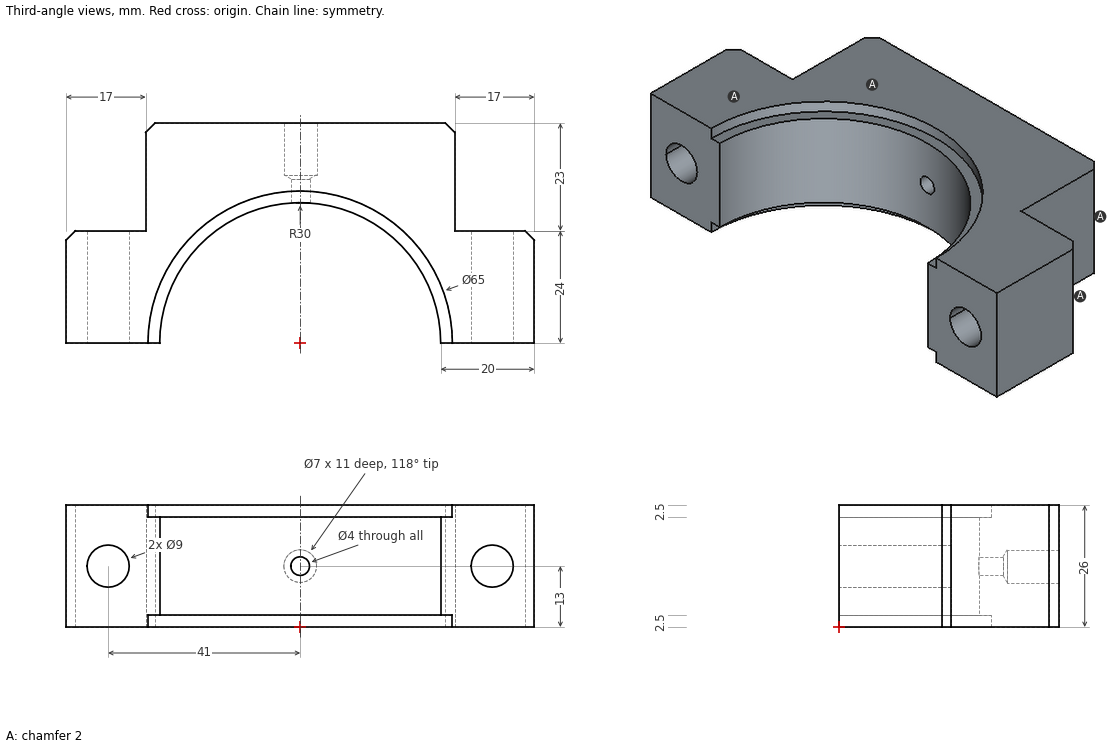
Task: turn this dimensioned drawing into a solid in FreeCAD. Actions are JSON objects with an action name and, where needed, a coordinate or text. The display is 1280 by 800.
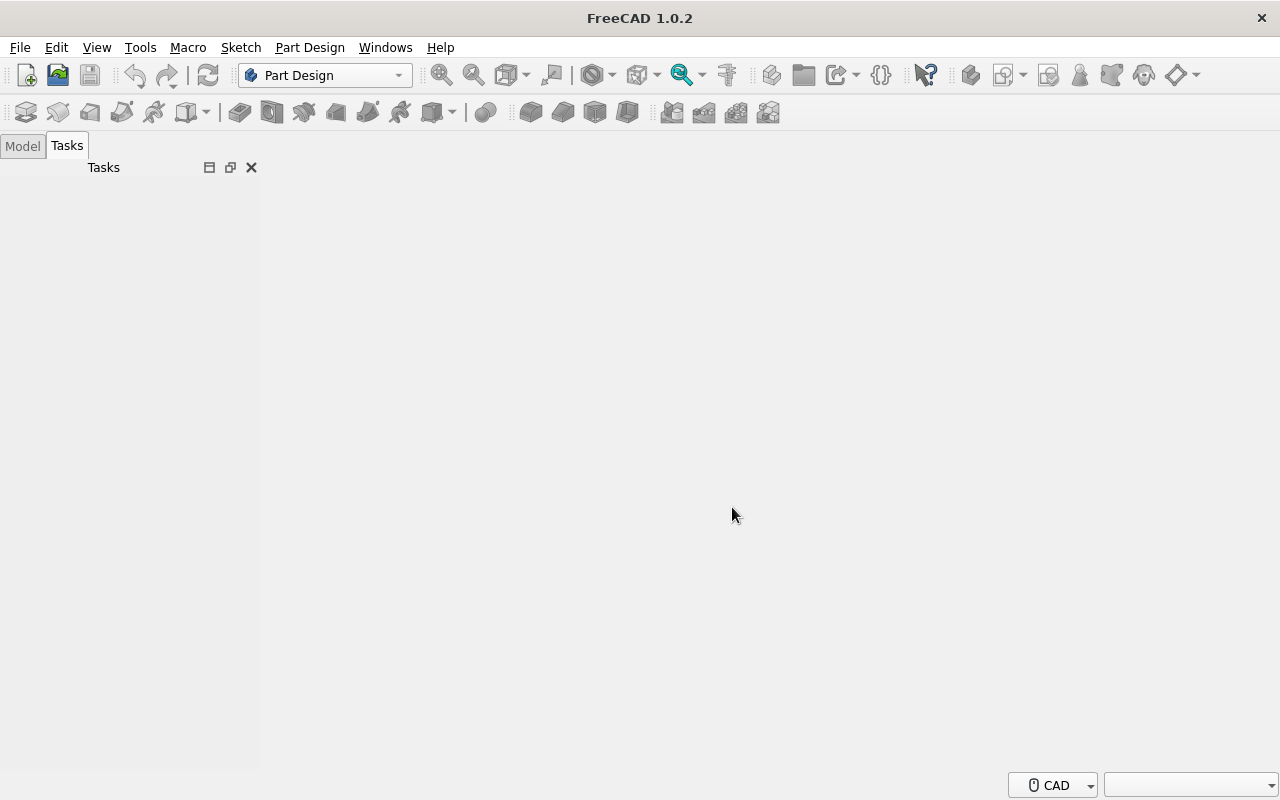
{"action": "key", "text": "ctrl+n"}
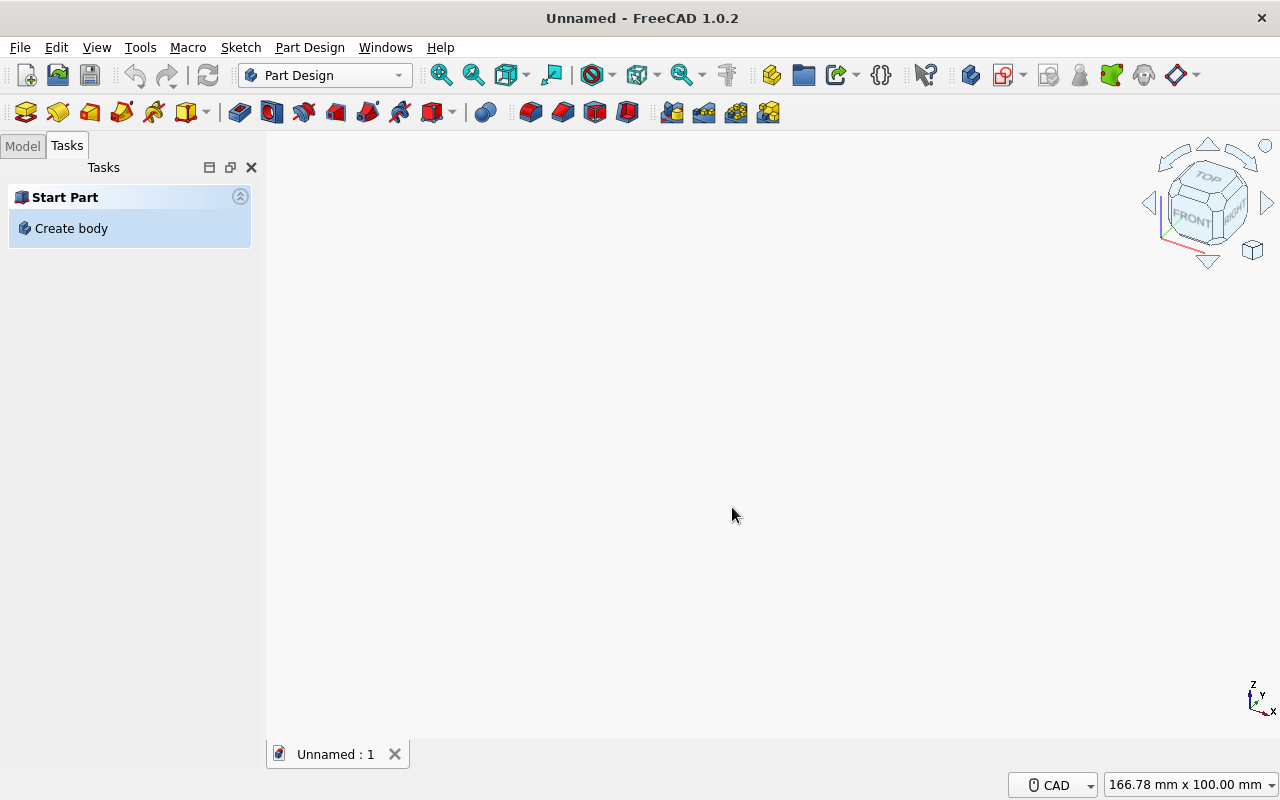
{"action": "left_click", "coordinate": [1004, 76]}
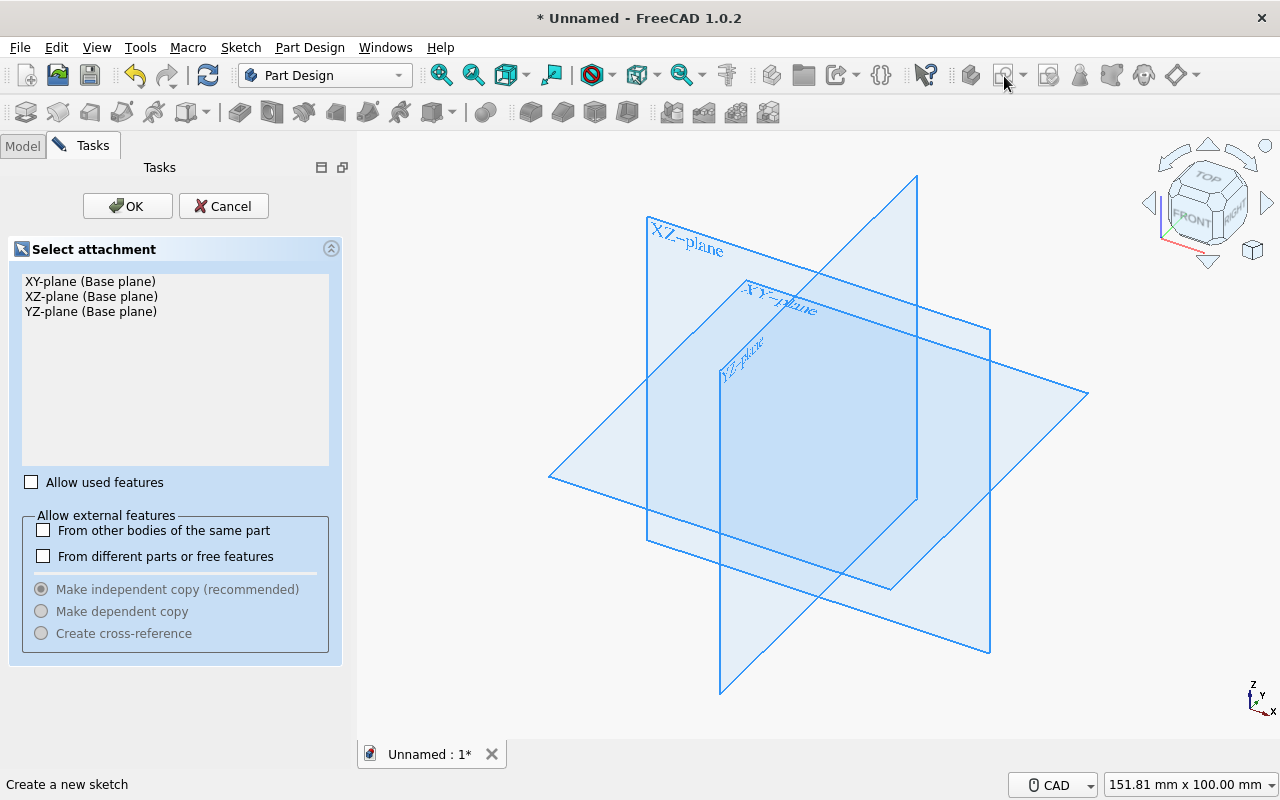
{"action": "left_click", "coordinate": [82, 282]}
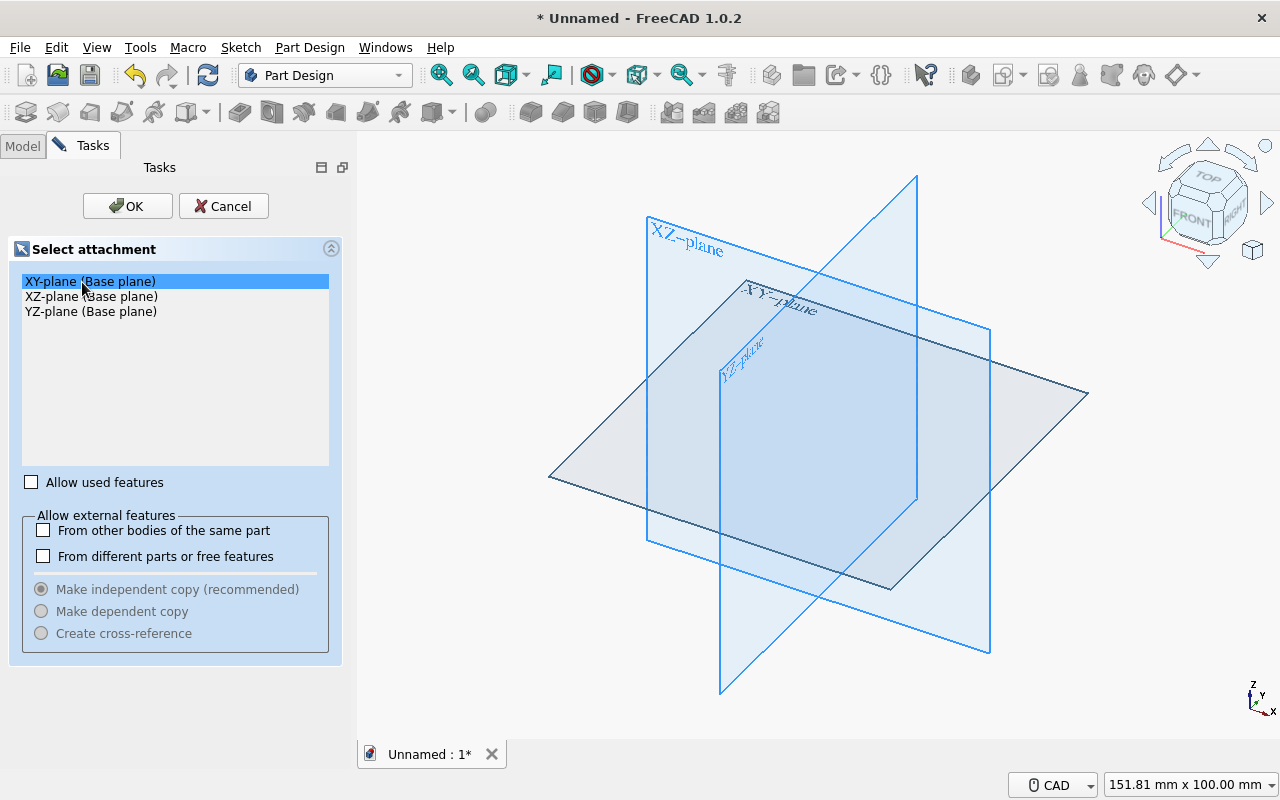
{"action": "left_click", "coordinate": [128, 206]}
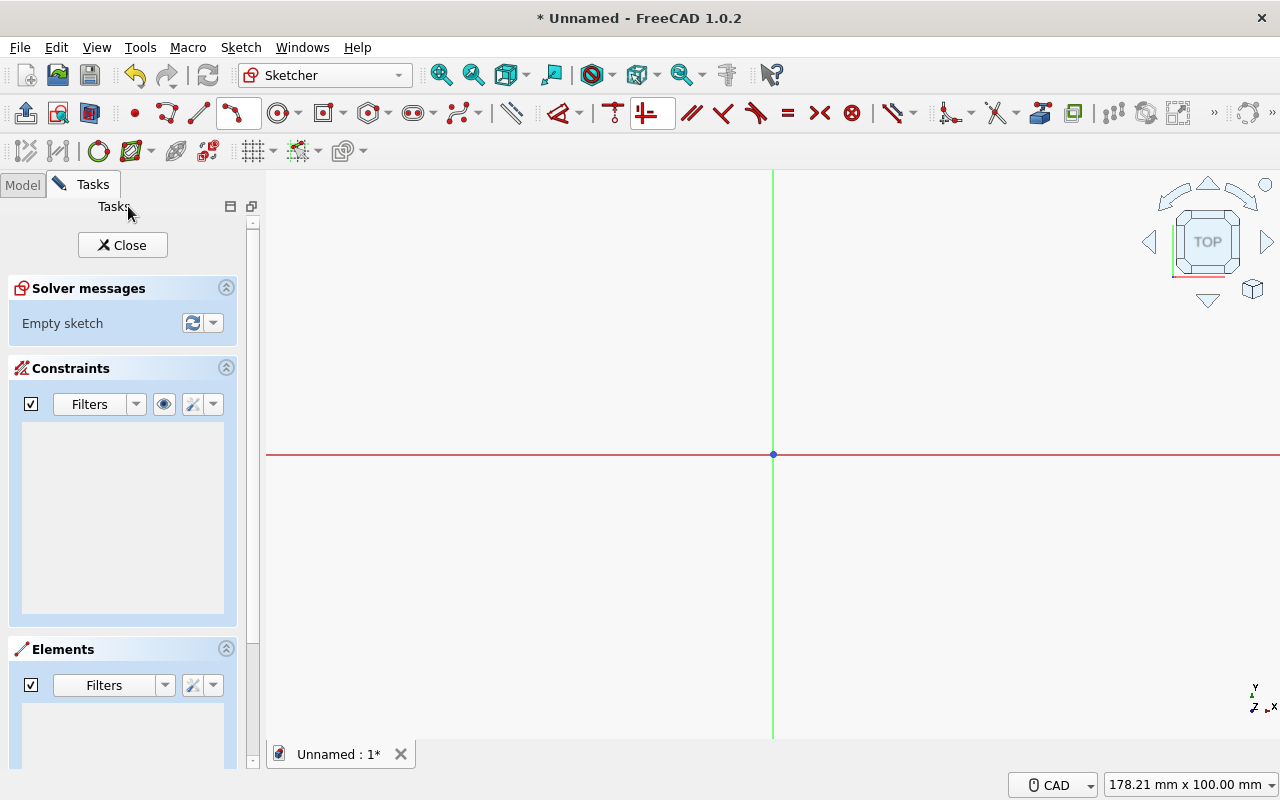
{"action": "scroll", "coordinate": [395, 711], "scroll_direction": "down", "scroll_amount": 1}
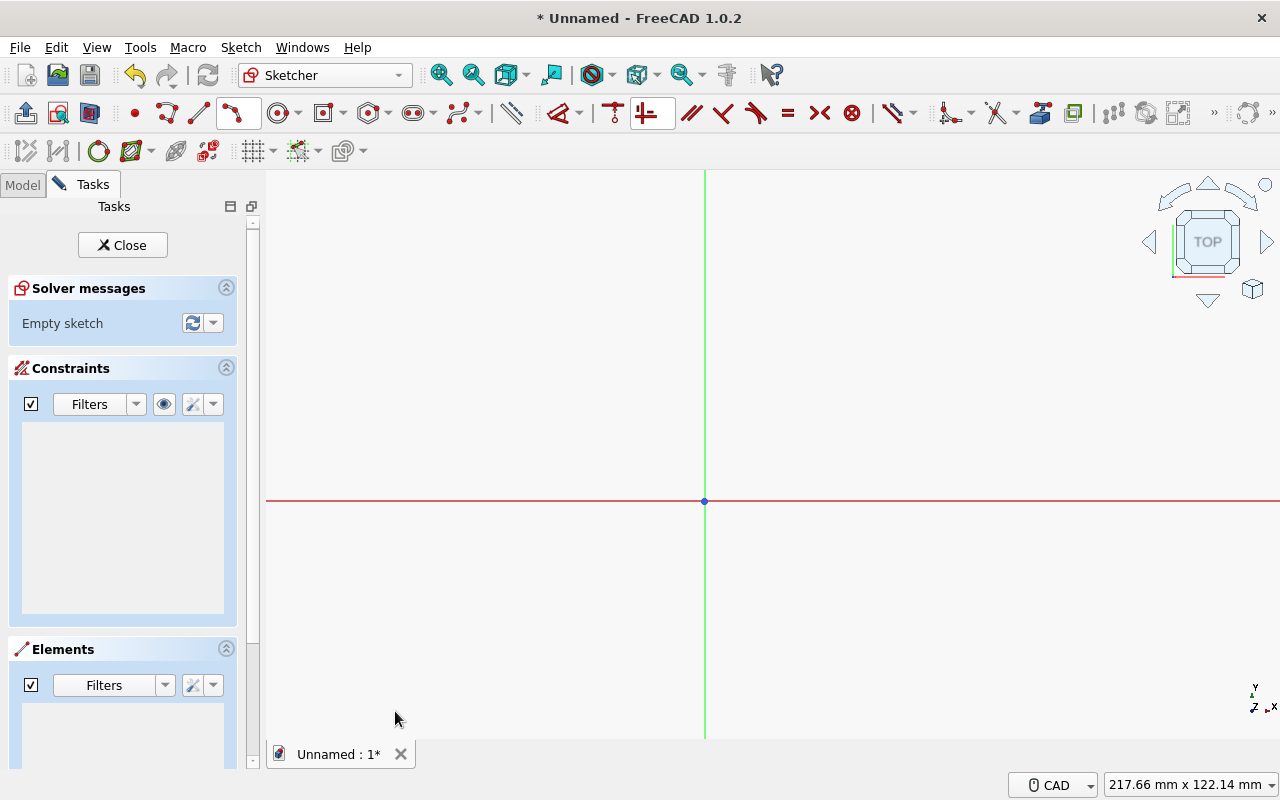
{"action": "left_click", "coordinate": [168, 114]}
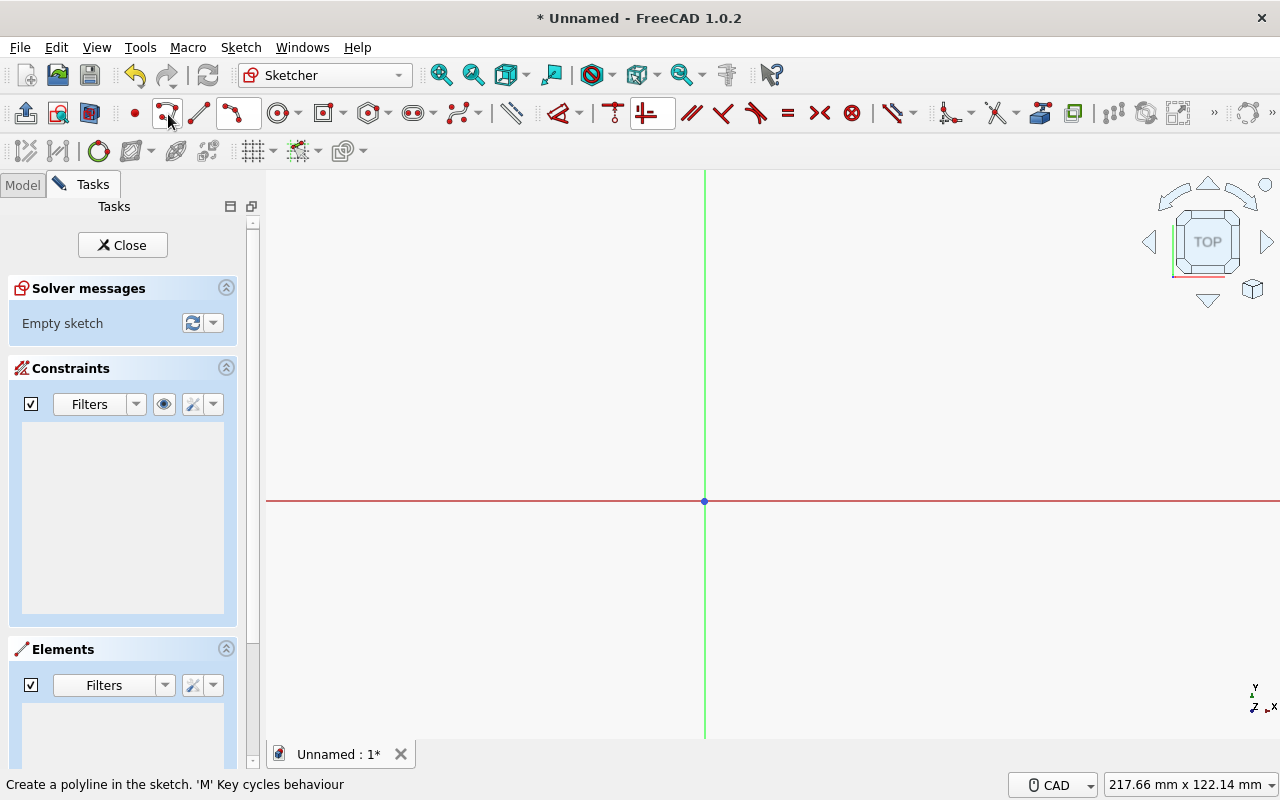
{"action": "left_click", "coordinate": [844, 501]}
{"action": "left_click", "coordinate": [937, 492]}
{"action": "left_click", "coordinate": [937, 389]}
{"action": "left_click", "coordinate": [858, 389]}
{"action": "left_click", "coordinate": [858, 282]}
{"action": "left_click", "coordinate": [551, 282]}
{"action": "left_click", "coordinate": [551, 389]}
{"action": "left_click", "coordinate": [472, 389]}
{"action": "left_click", "coordinate": [472, 501]}
{"action": "left_click", "coordinate": [565, 492]}
{"action": "right_click", "coordinate": [565, 492]}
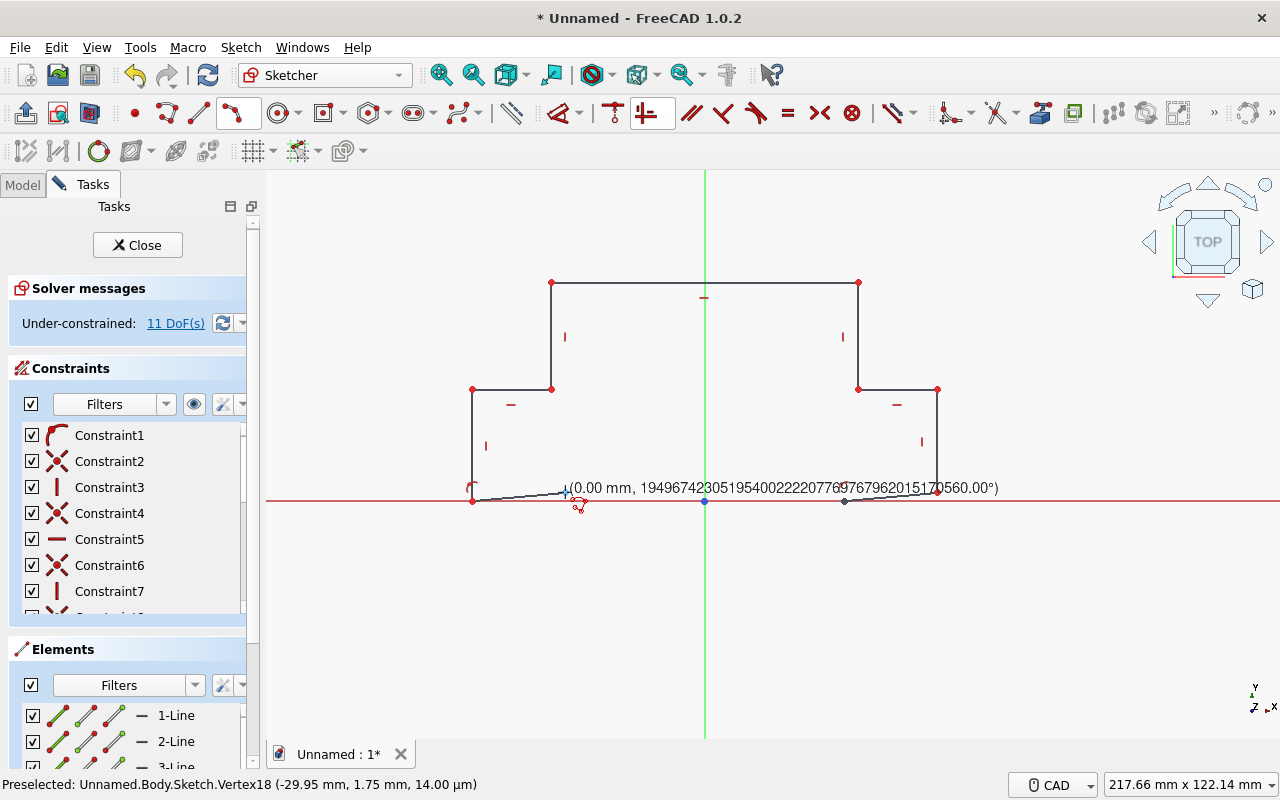
{"action": "key", "text": "g 3 a"}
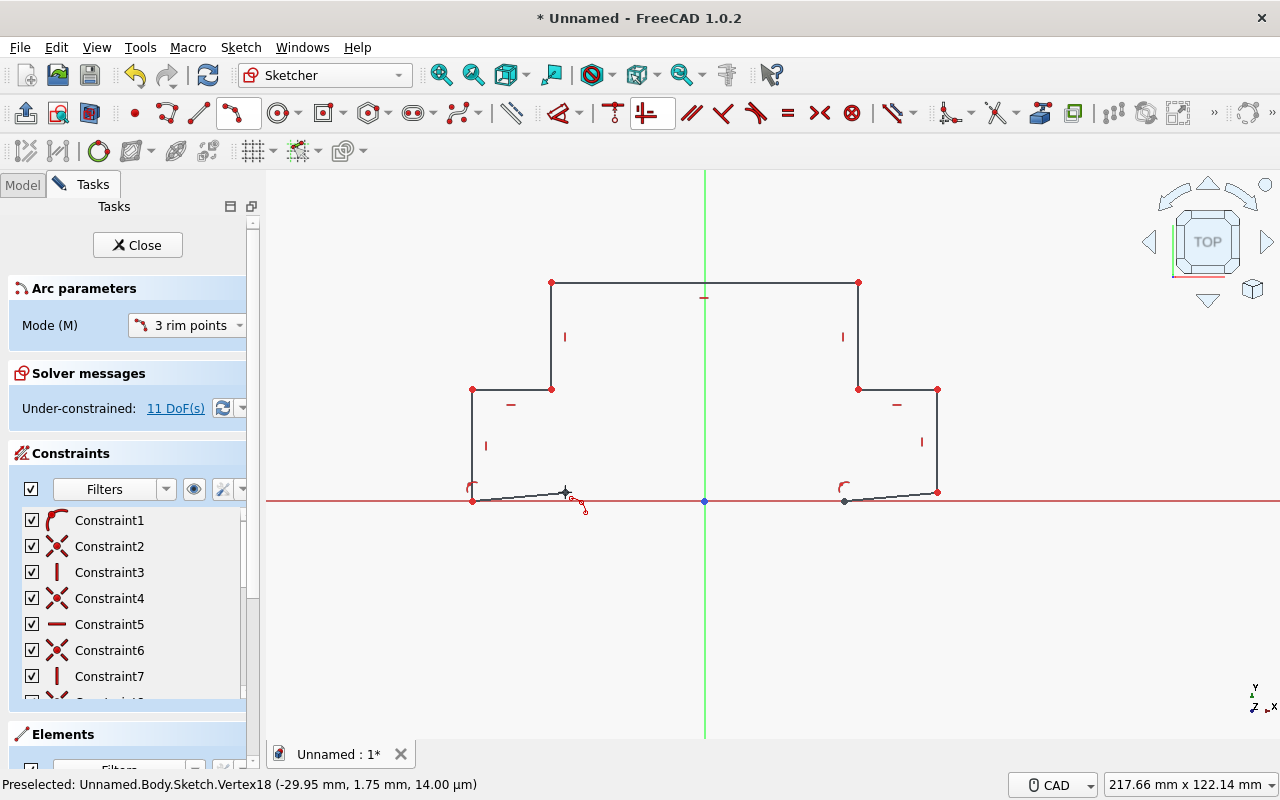
{"action": "left_click", "coordinate": [565, 493]}
{"action": "left_click", "coordinate": [844, 501]}
{"action": "left_click", "coordinate": [748, 368]}
{"action": "key", "text": "Escape"}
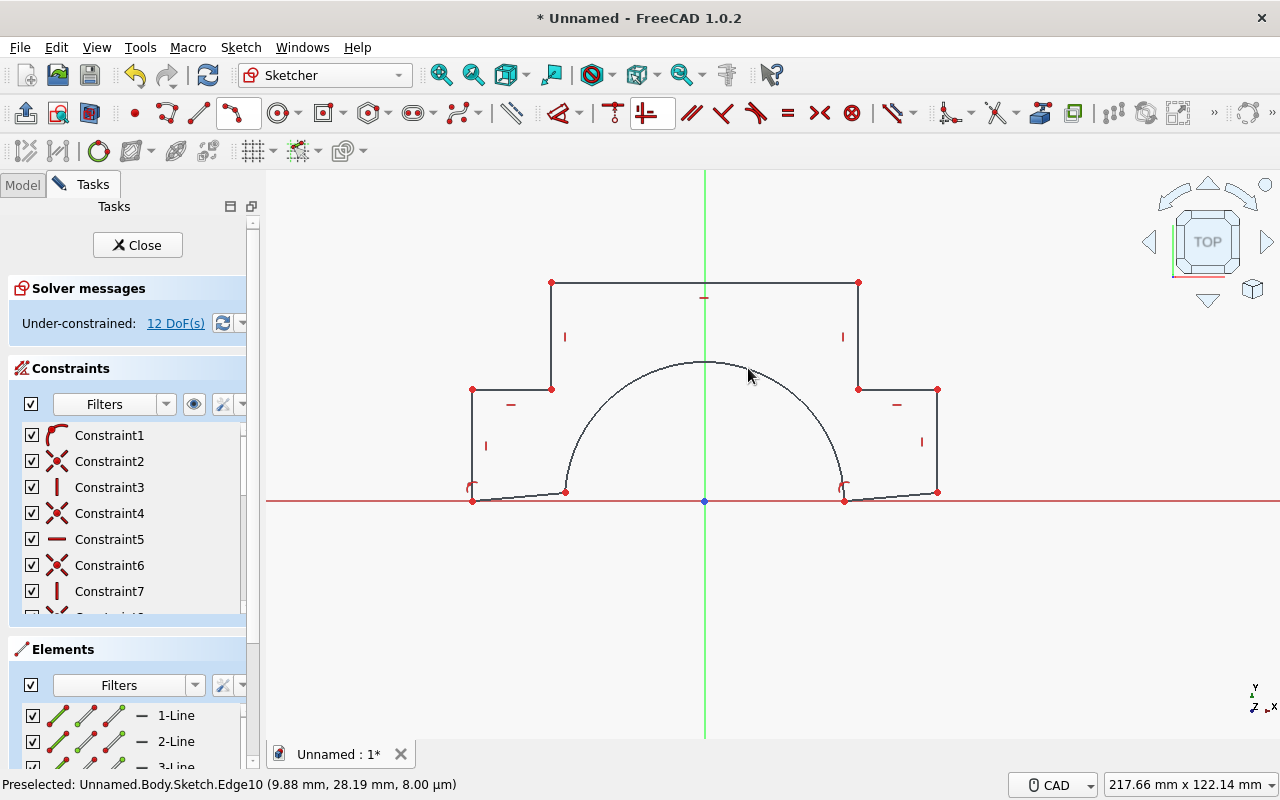
{"action": "left_click", "coordinate": [872, 499]}